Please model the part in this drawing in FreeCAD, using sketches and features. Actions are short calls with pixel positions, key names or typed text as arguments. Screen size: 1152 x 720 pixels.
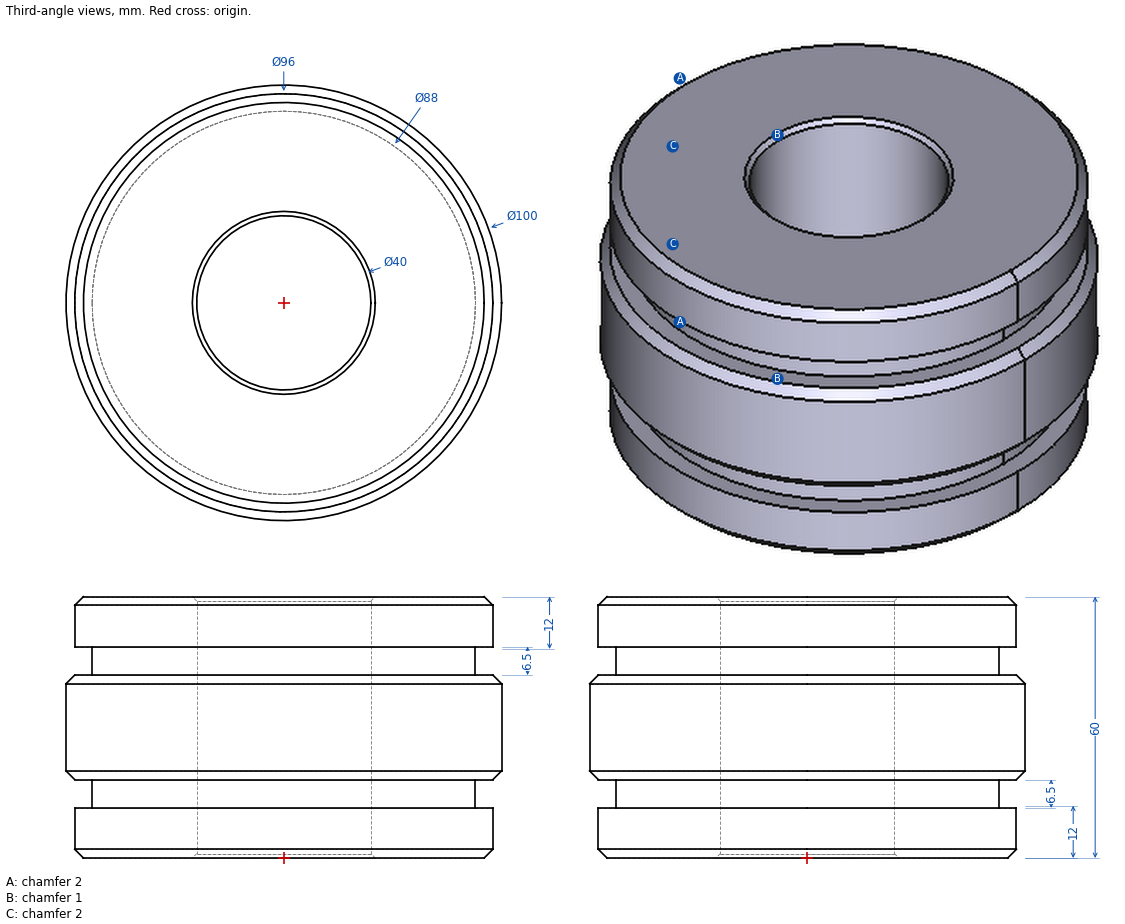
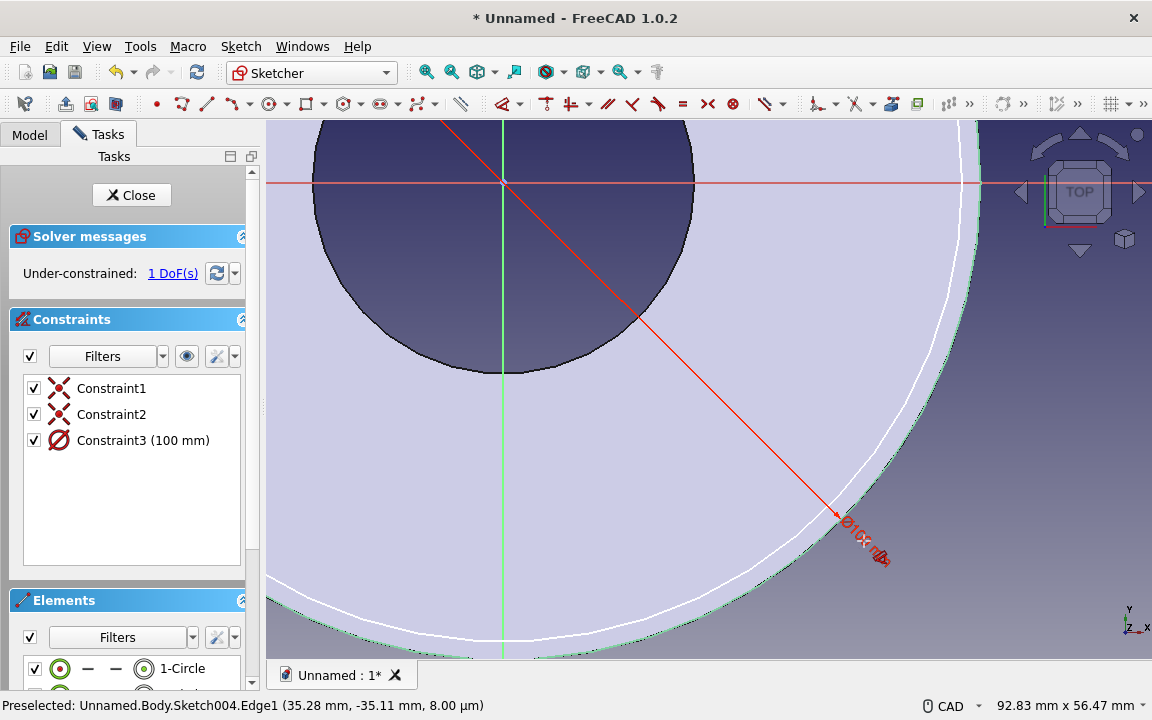
click(829, 506)
click(975, 319)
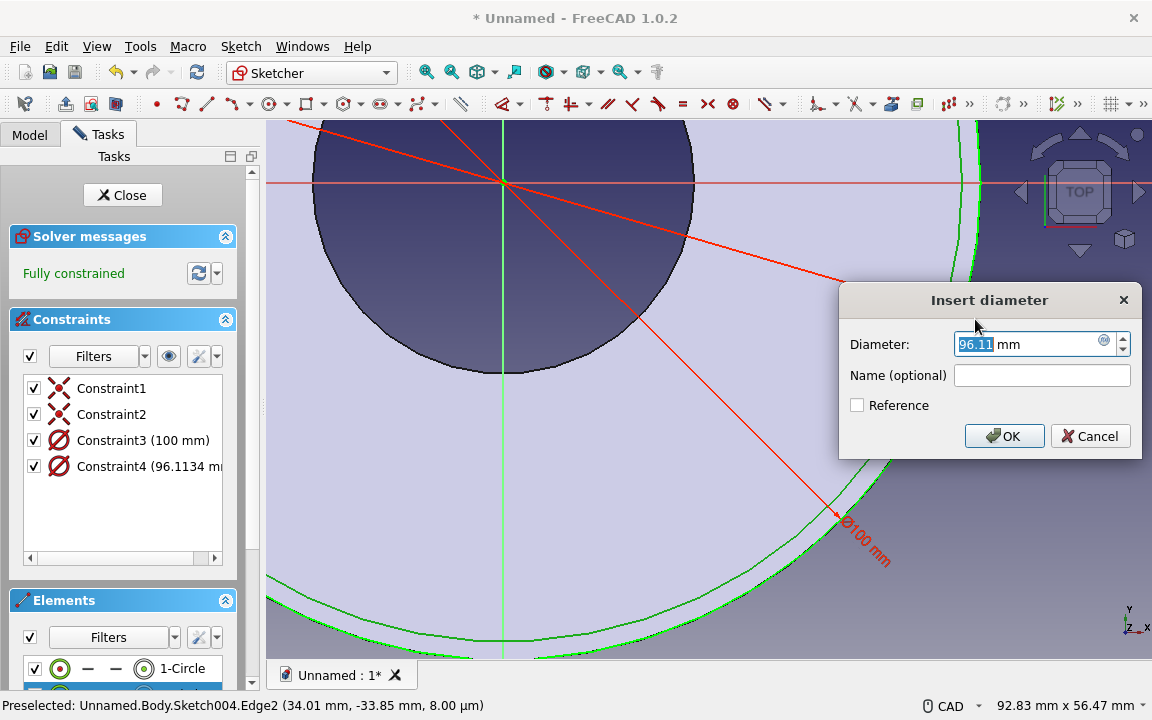
text(96)
key(Return)
key(Escape)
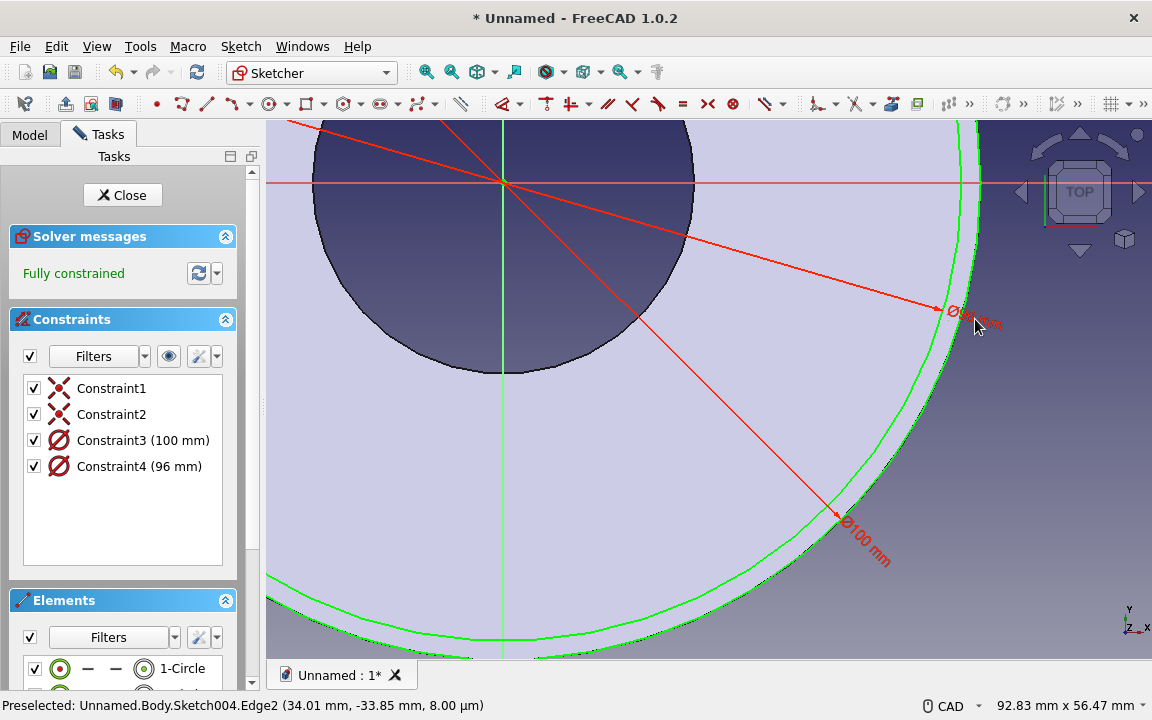
click(123, 195)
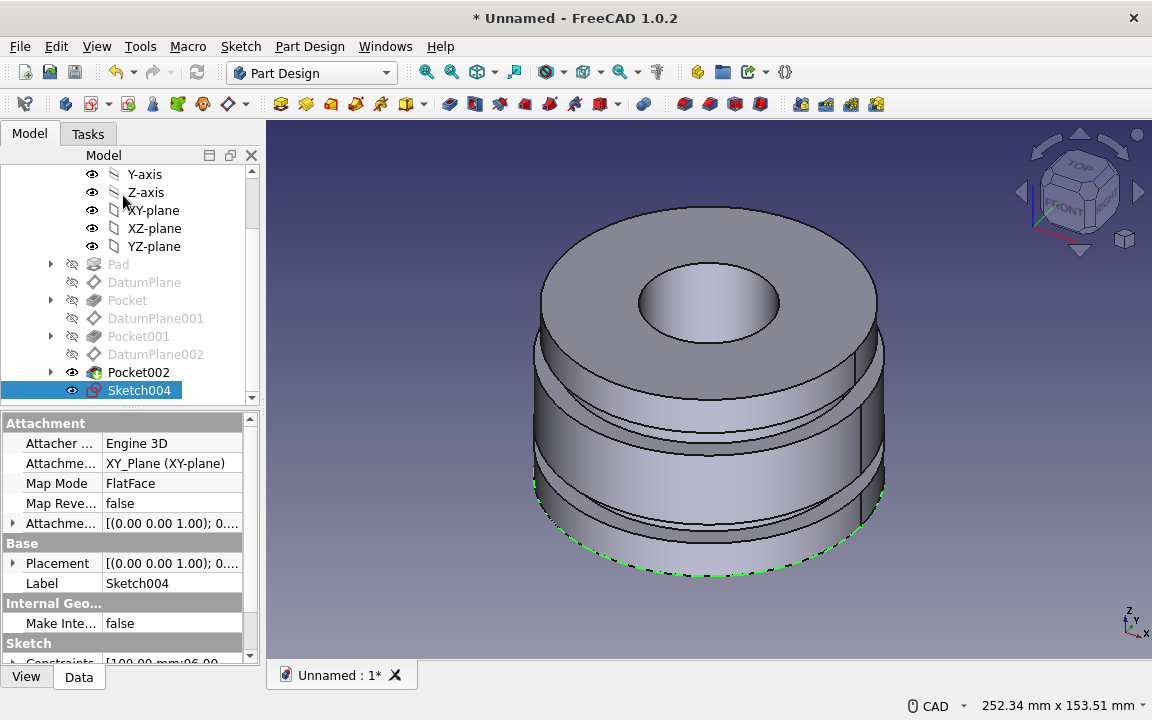
click(450, 104)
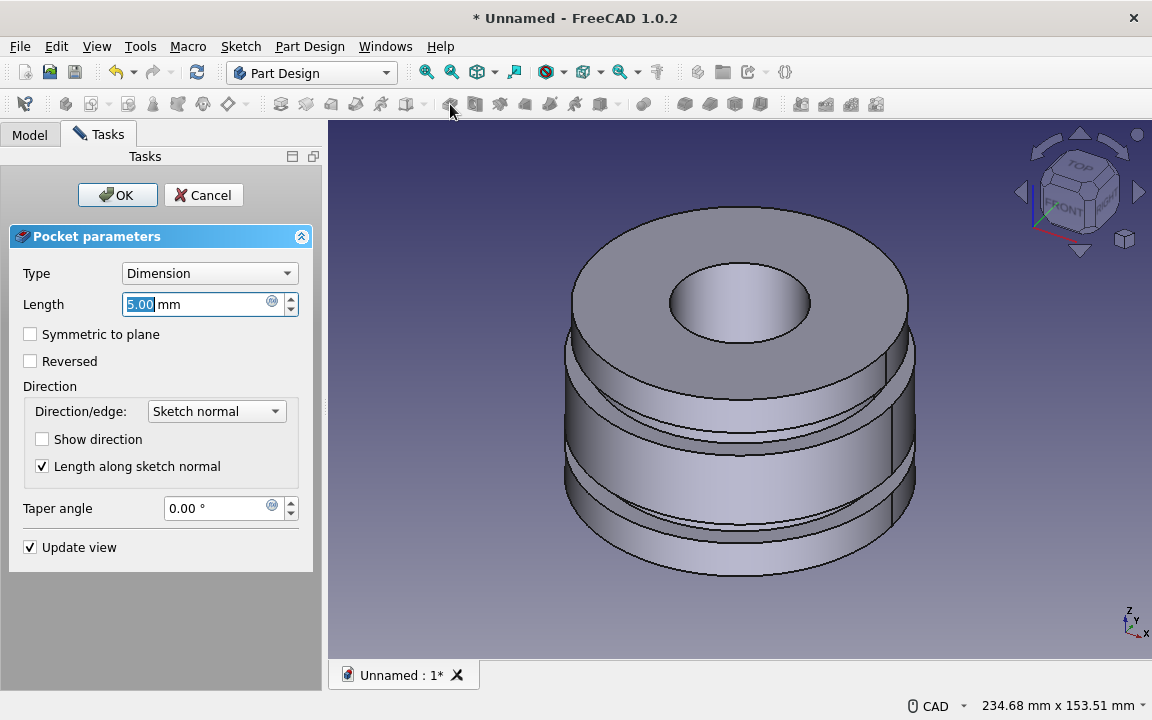
text(12)
key(Tab)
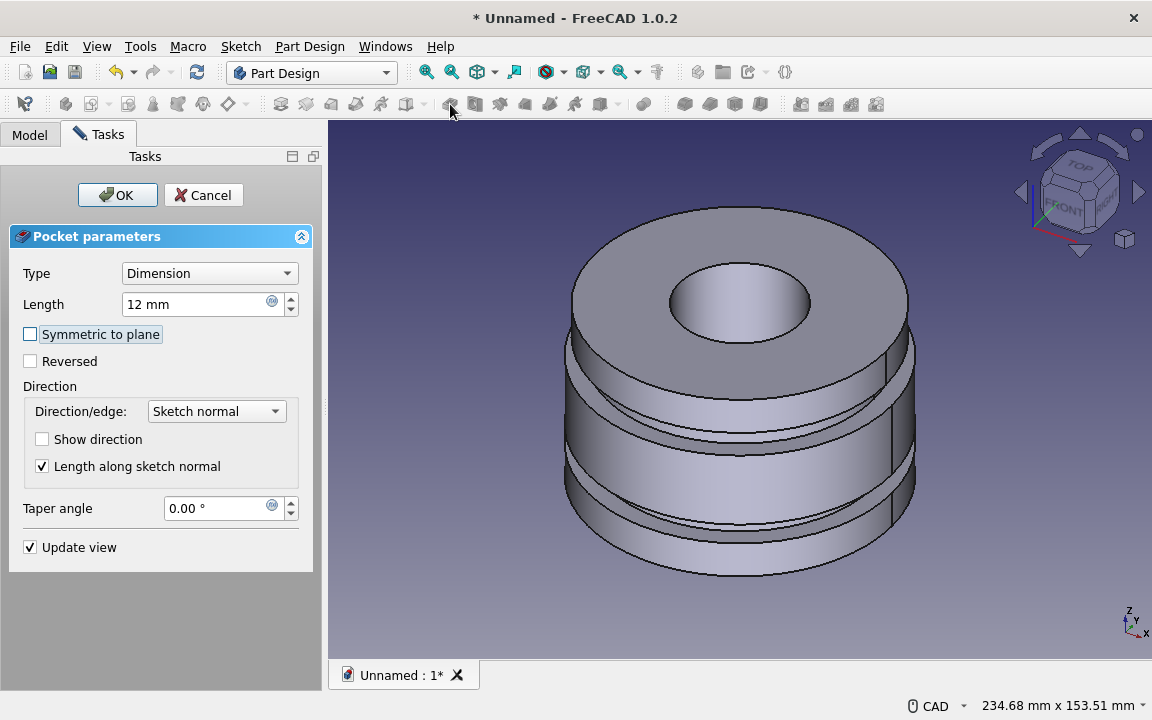
click(31, 361)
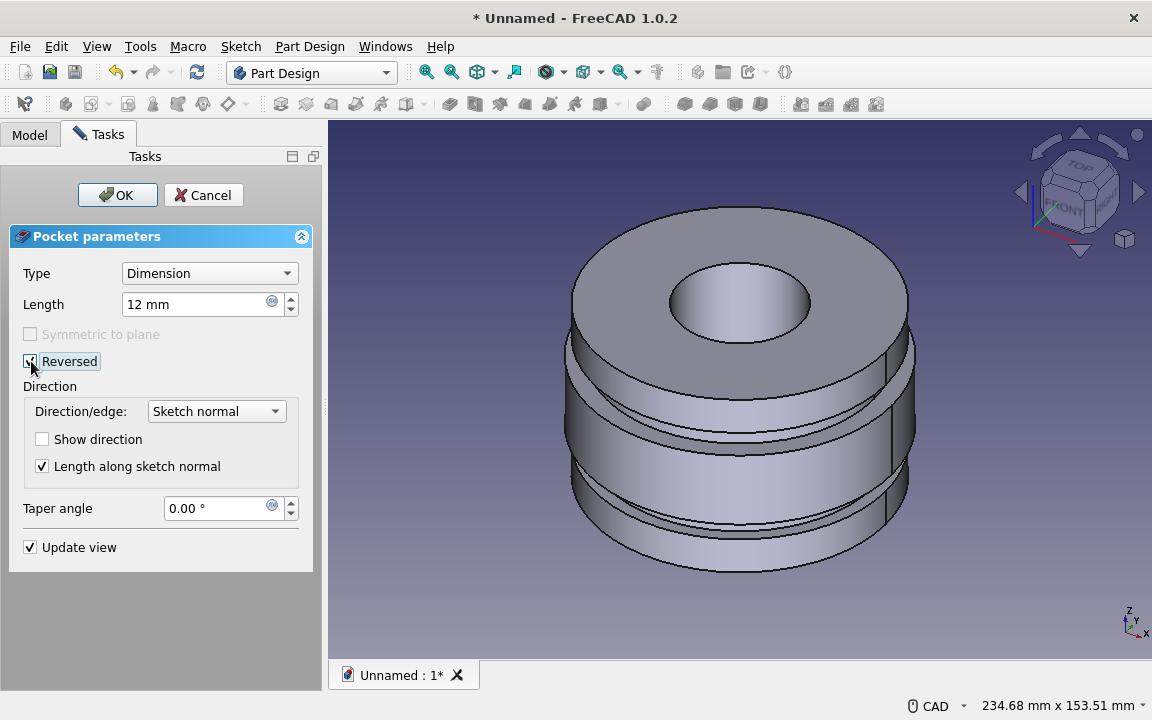
click(118, 195)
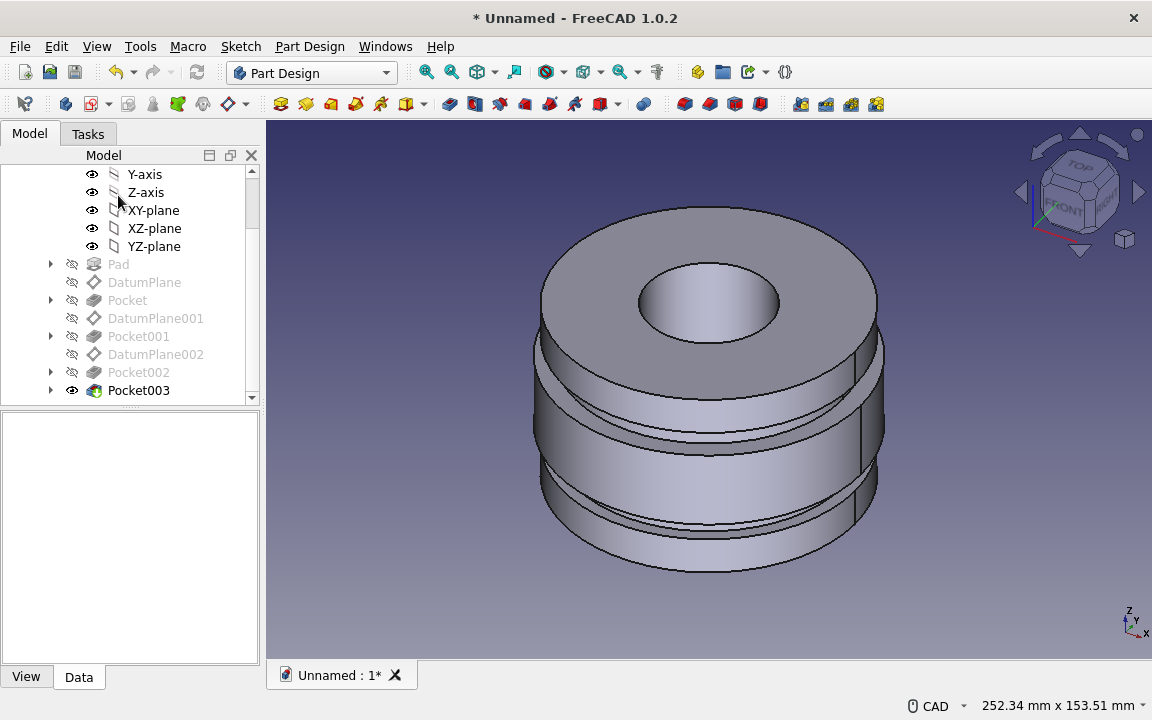
click(541, 312)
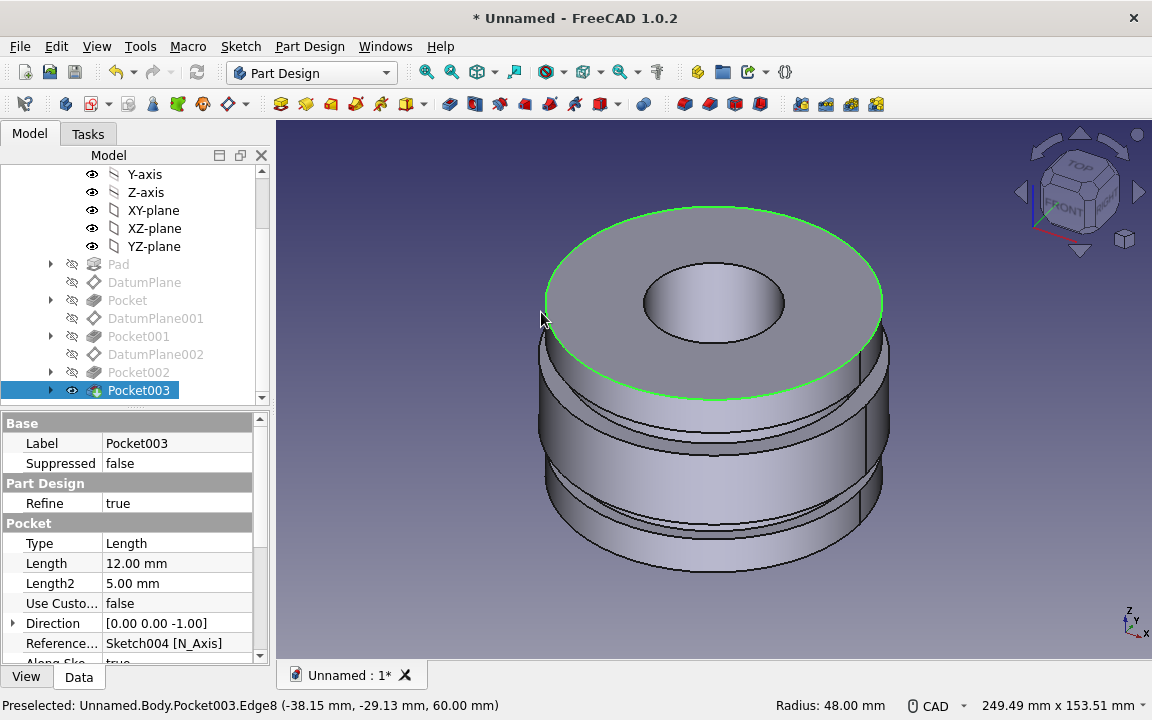
key(0)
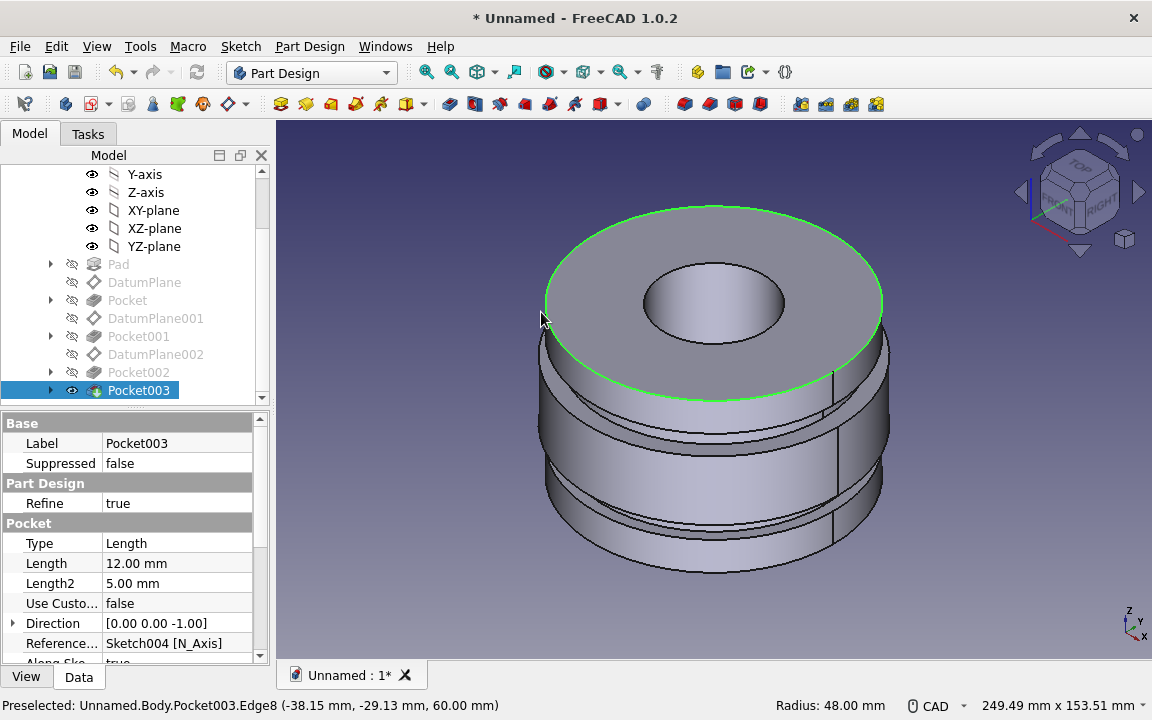
key(2)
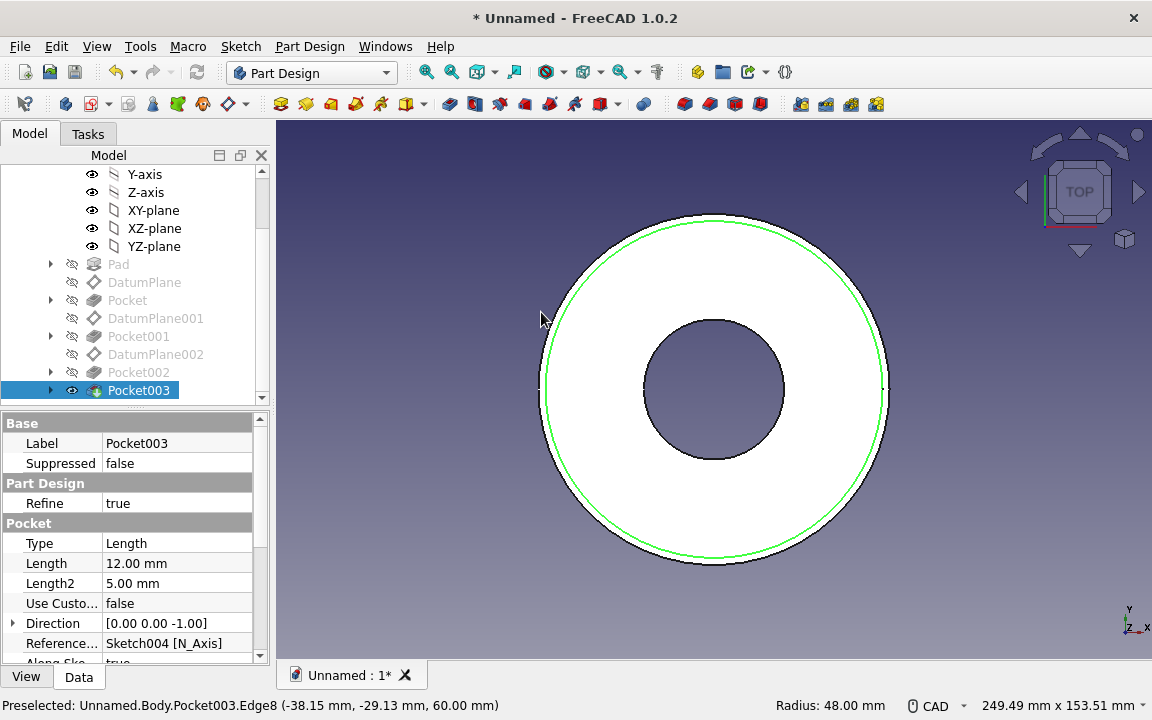
key(1)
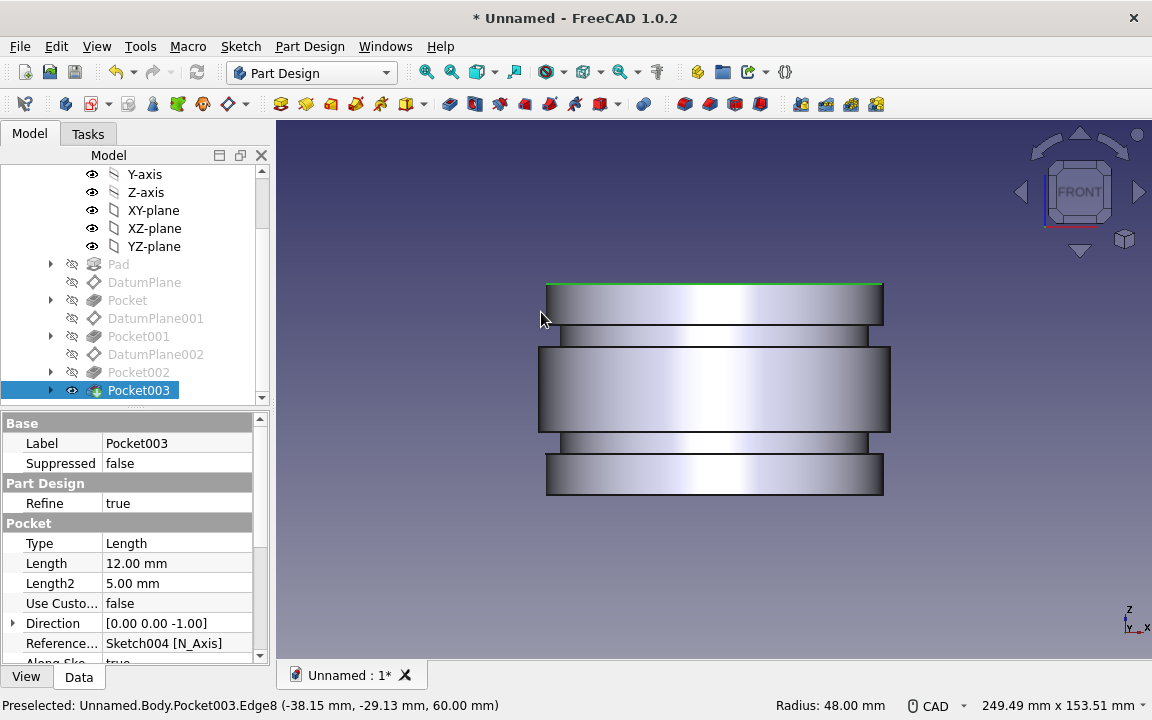
click(427, 72)